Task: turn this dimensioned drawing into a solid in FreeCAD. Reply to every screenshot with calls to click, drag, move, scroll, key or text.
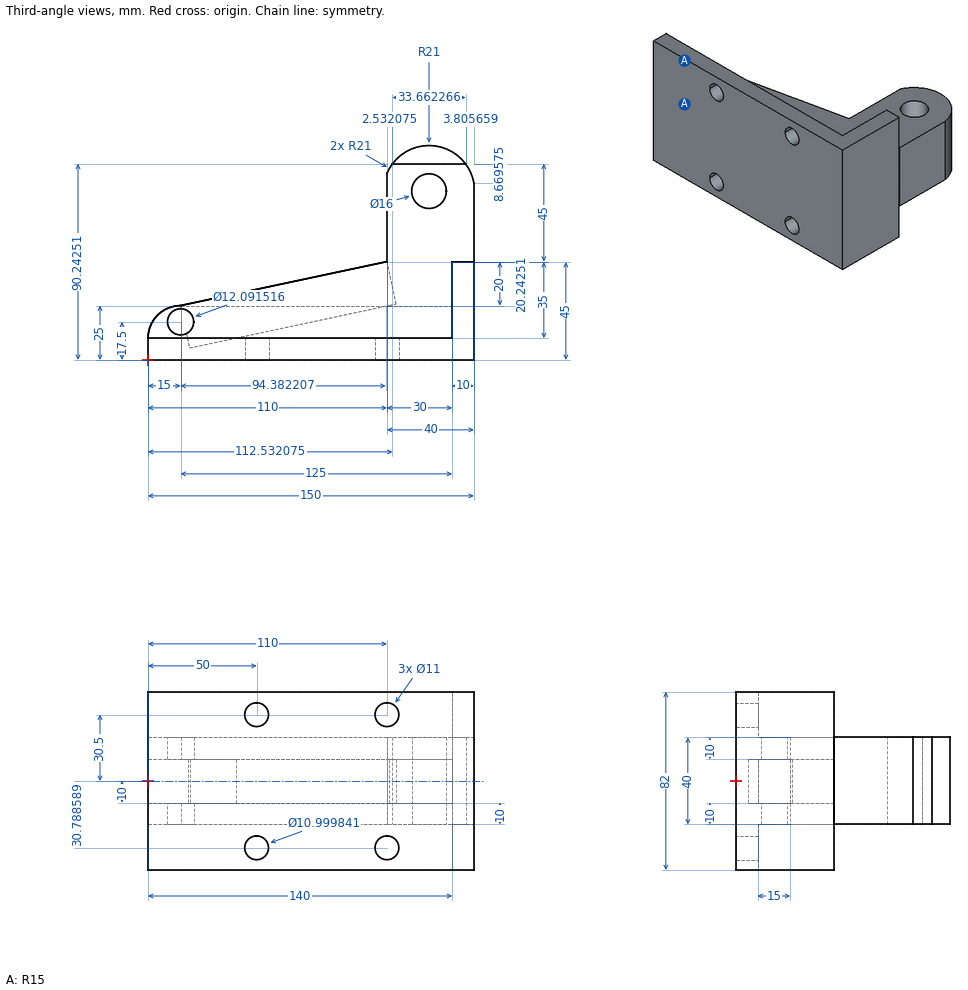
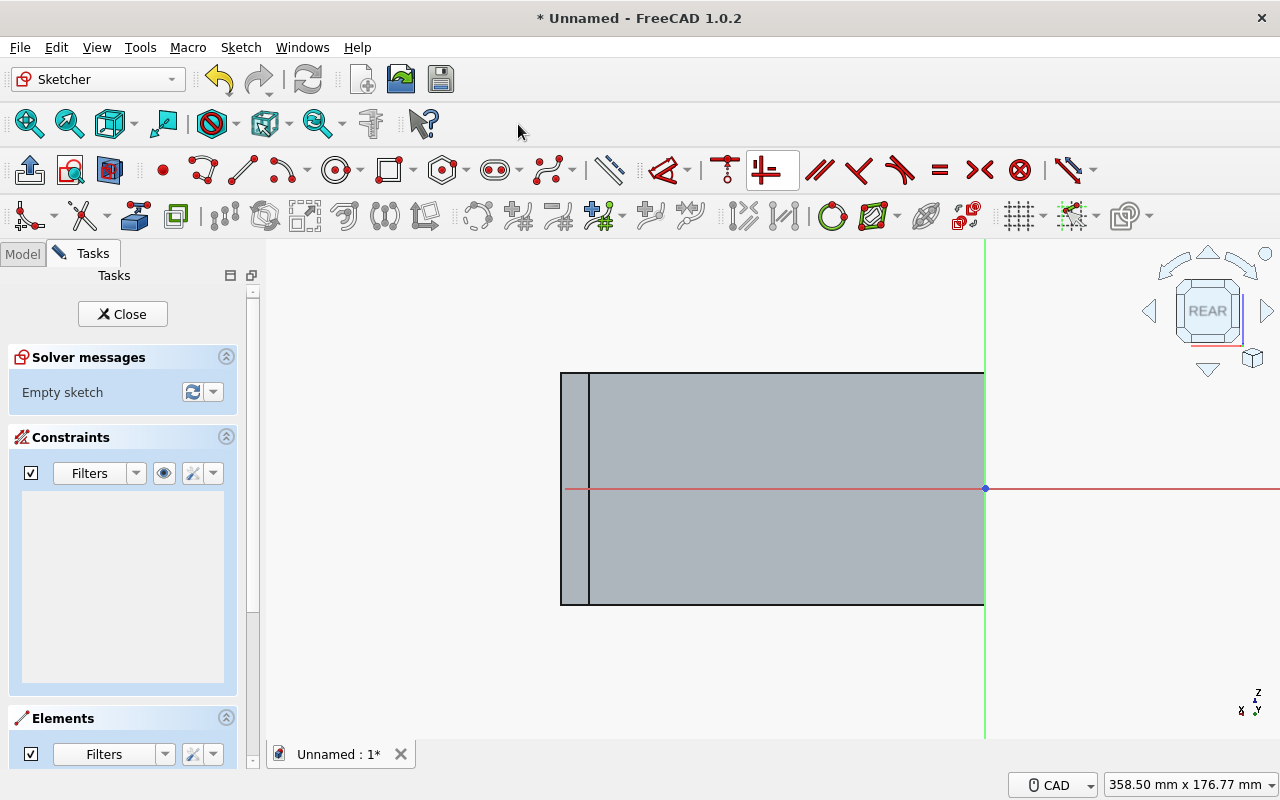
scroll(955, 489, up, 2)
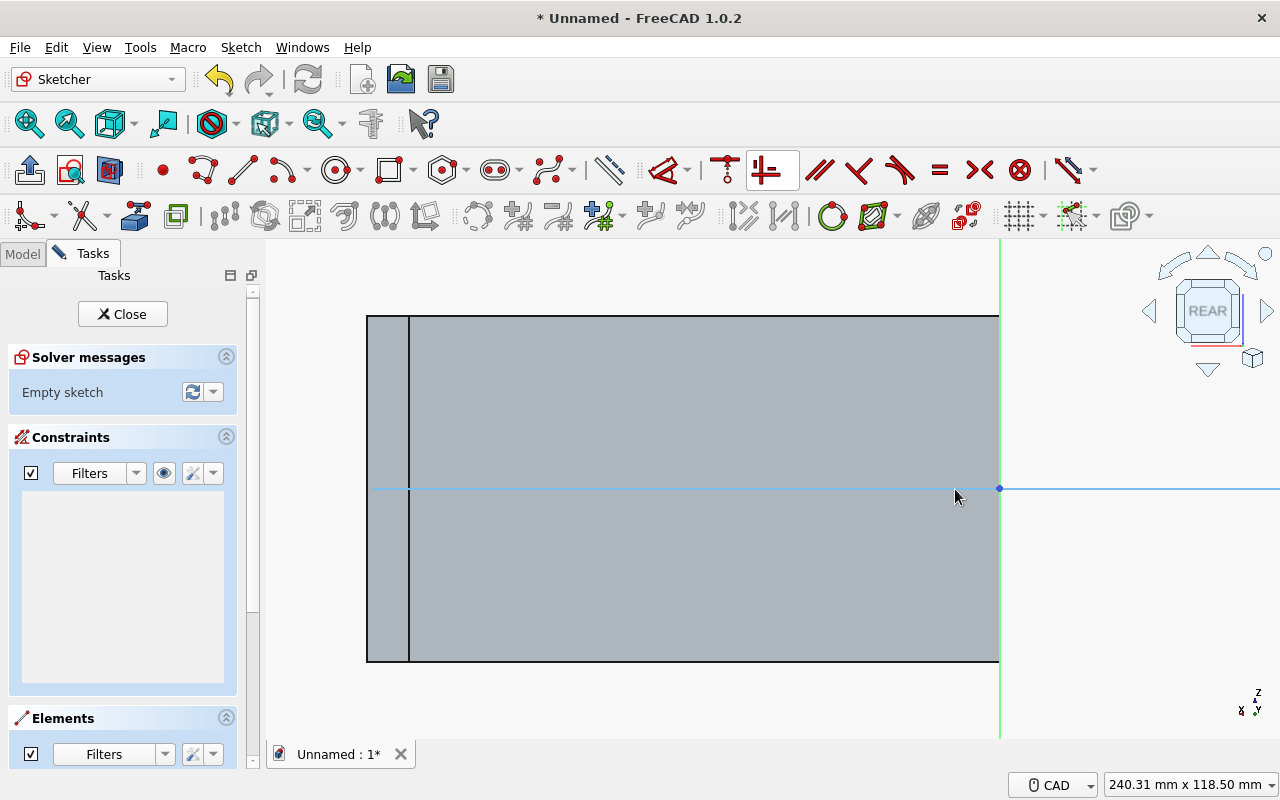
key(g)
key(r)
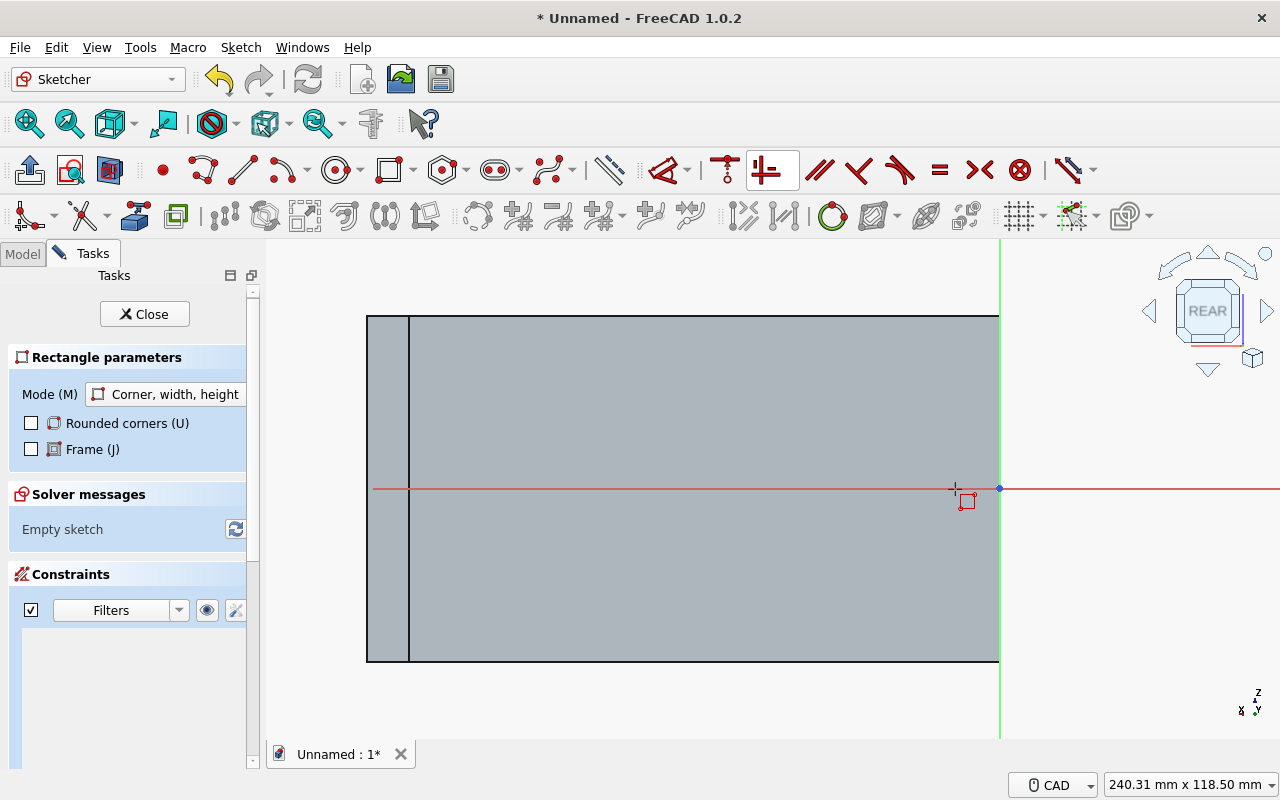
click(409, 531)
click(1000, 573)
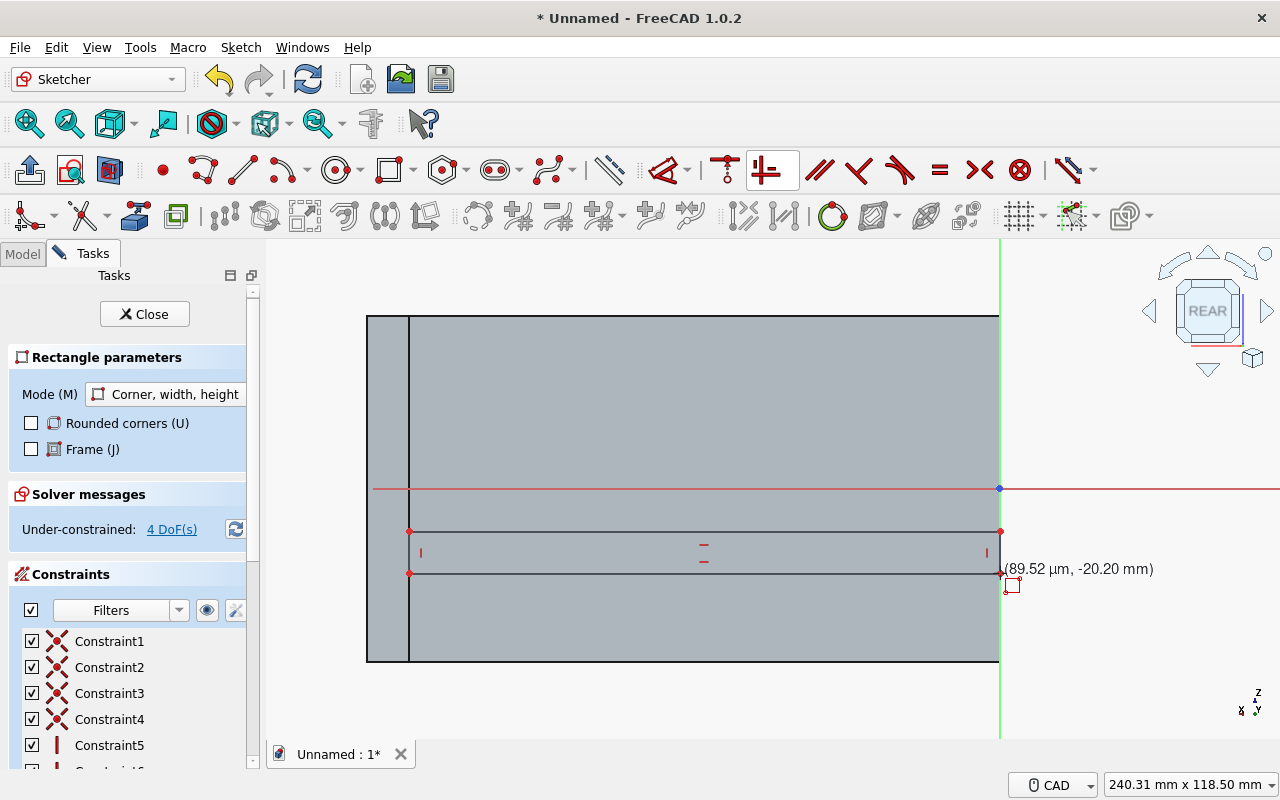
click(409, 404)
click(1000, 447)
key(Escape)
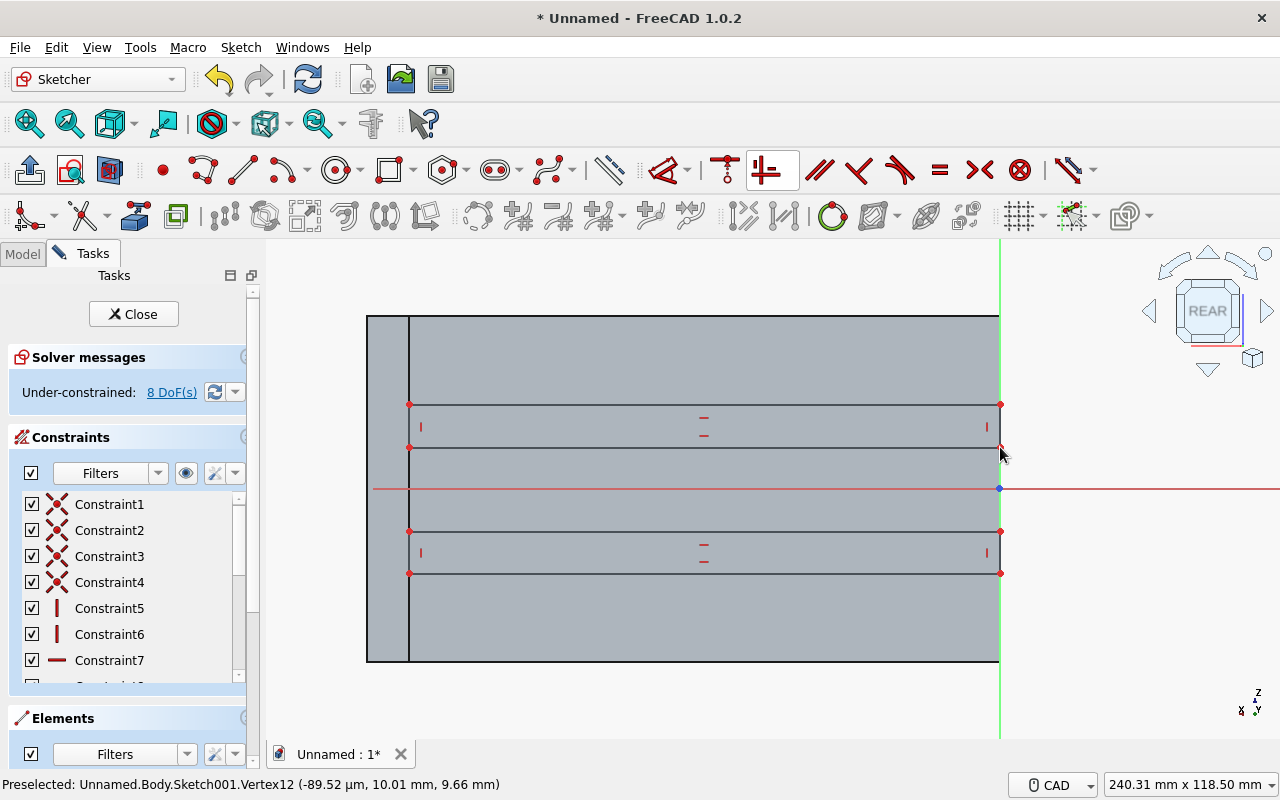
click(409, 574)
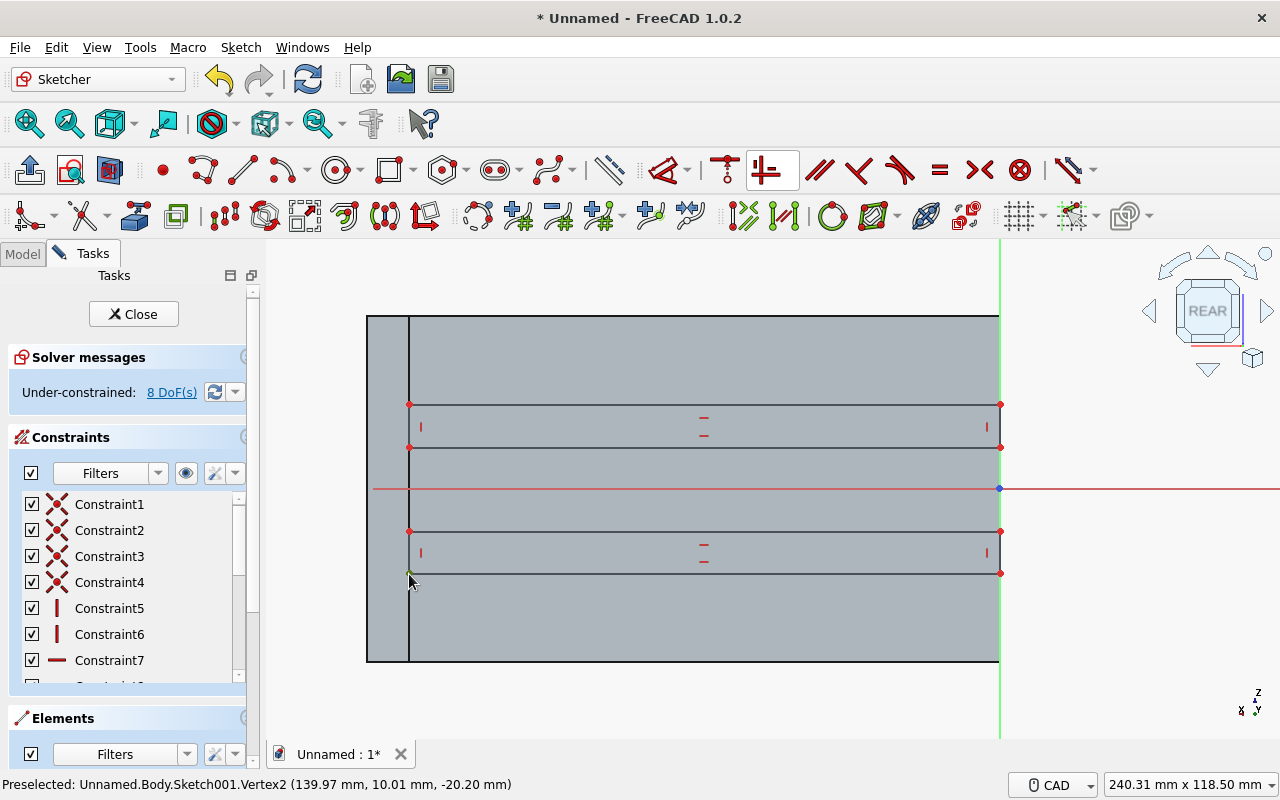
click(409, 405)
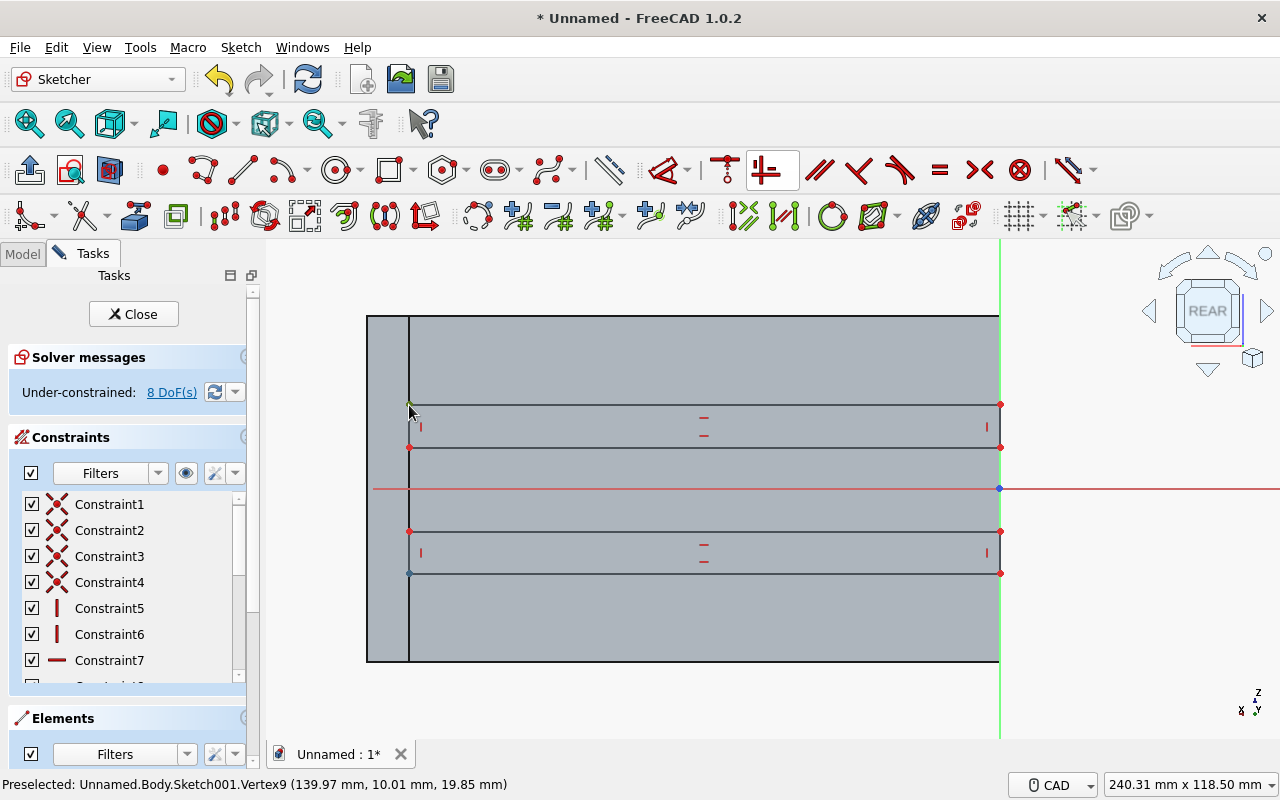
click(411, 489)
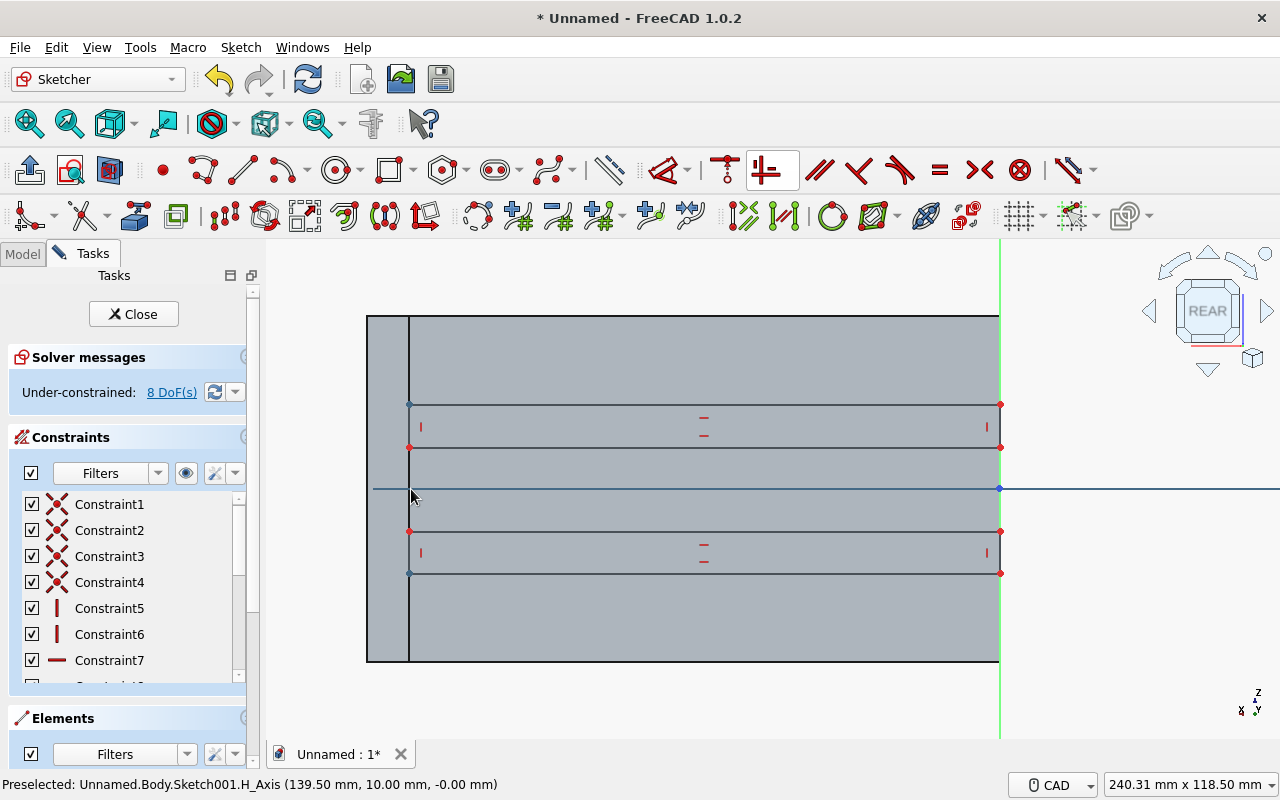
key(s)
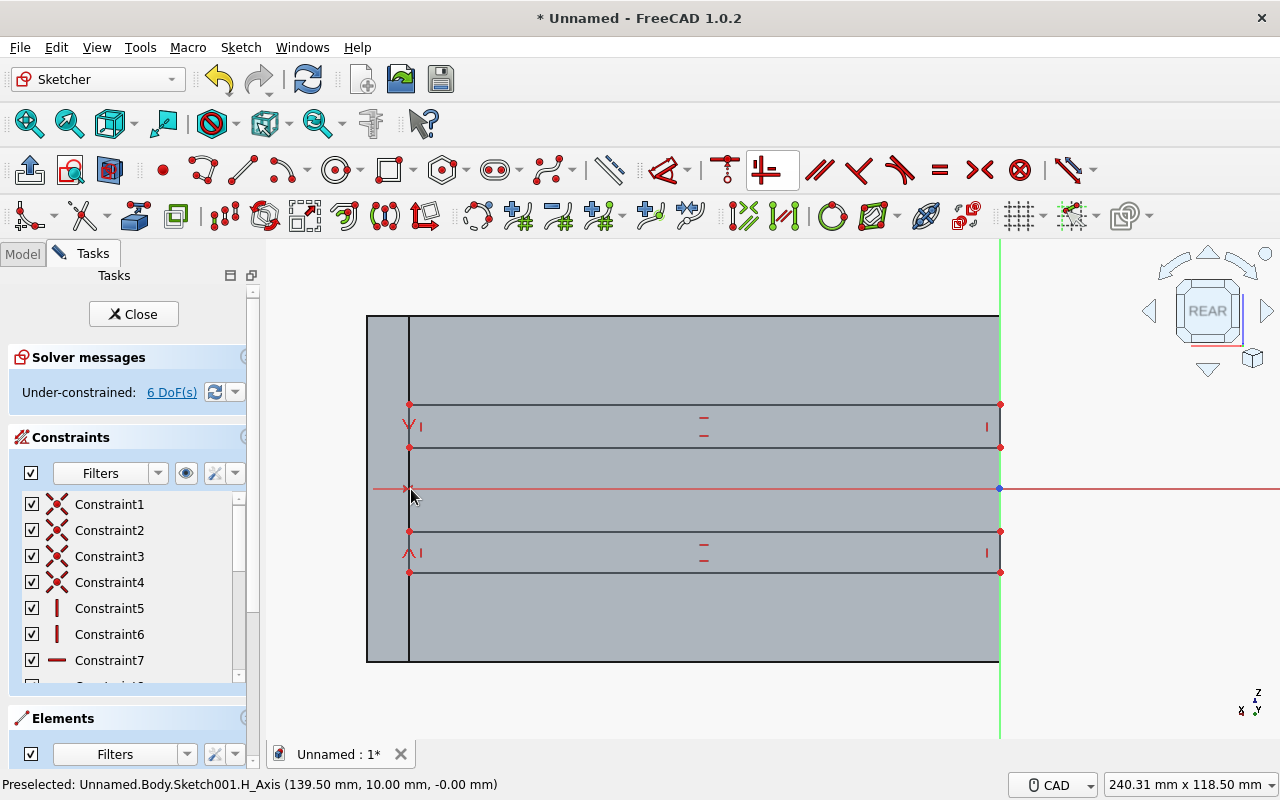
click(1000, 532)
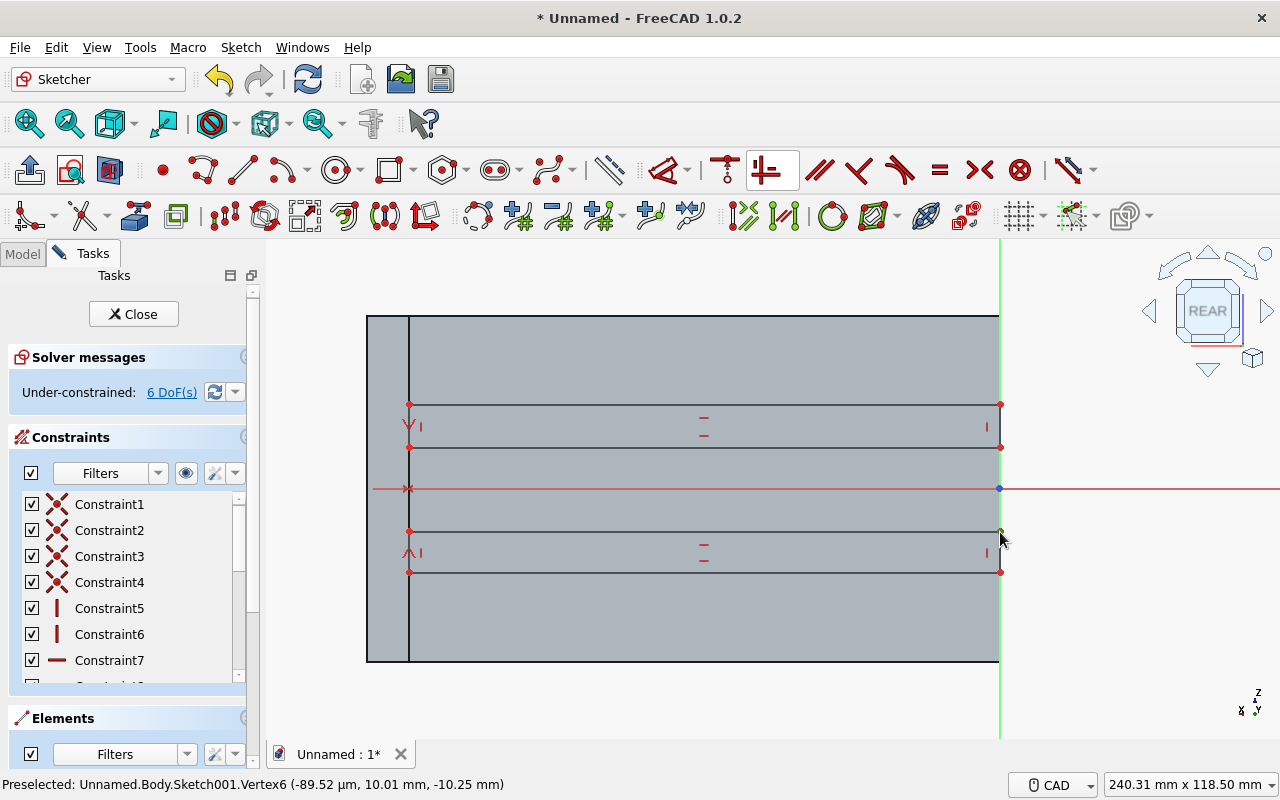
click(1000, 448)